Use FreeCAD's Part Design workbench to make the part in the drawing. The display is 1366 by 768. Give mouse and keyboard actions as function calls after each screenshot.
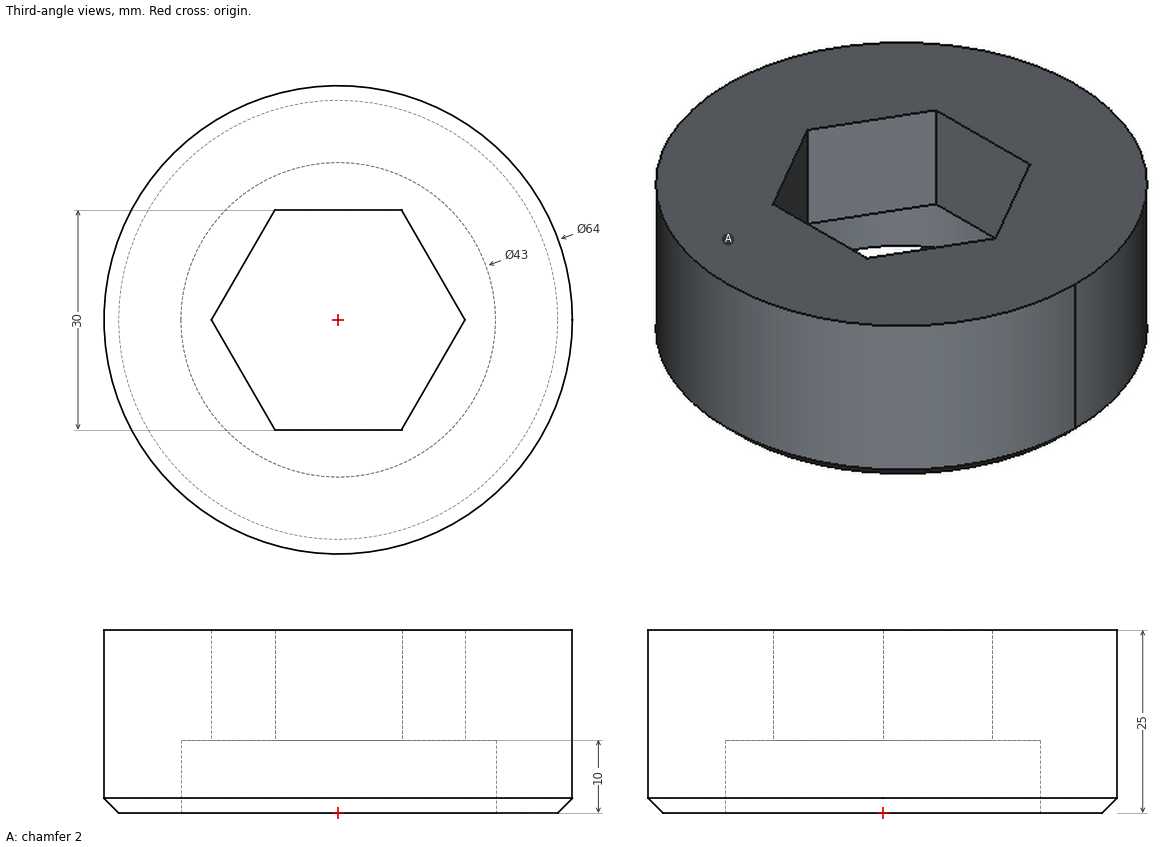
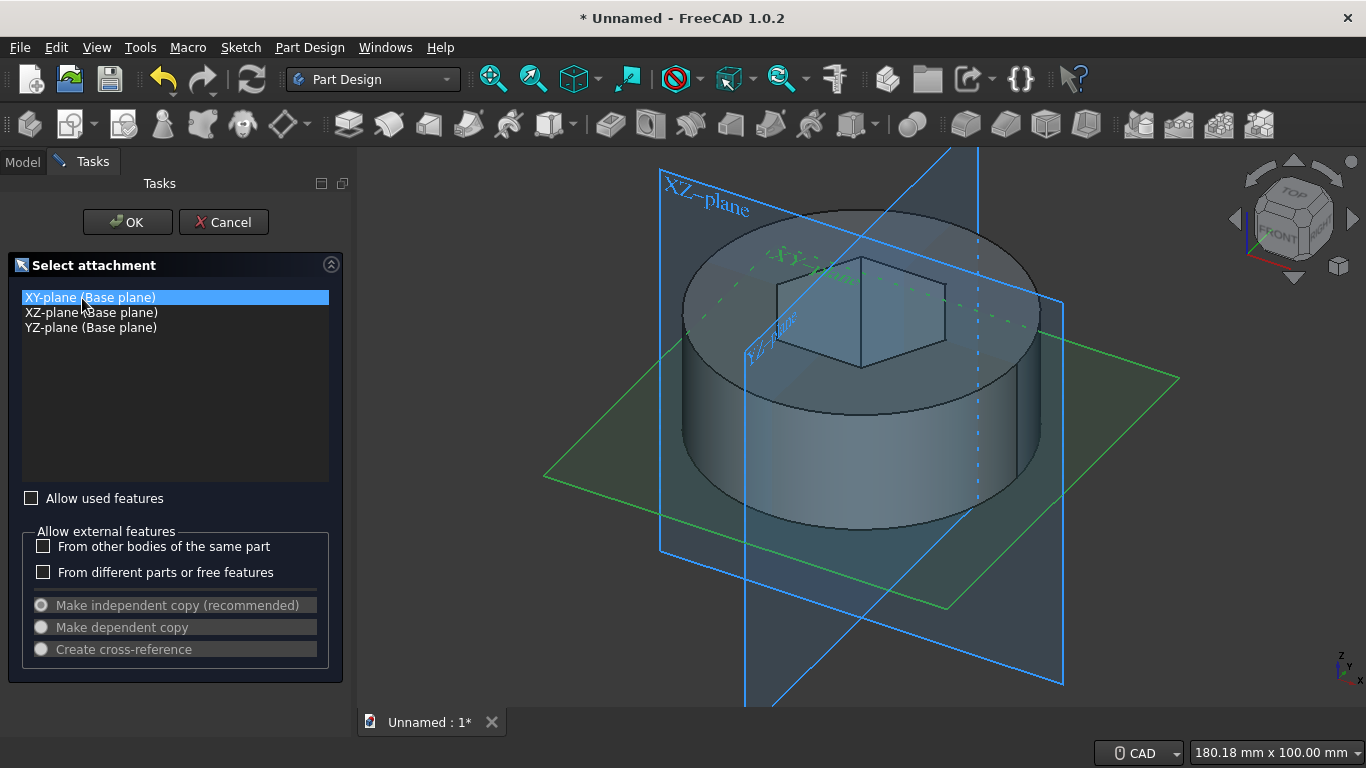
click(128, 222)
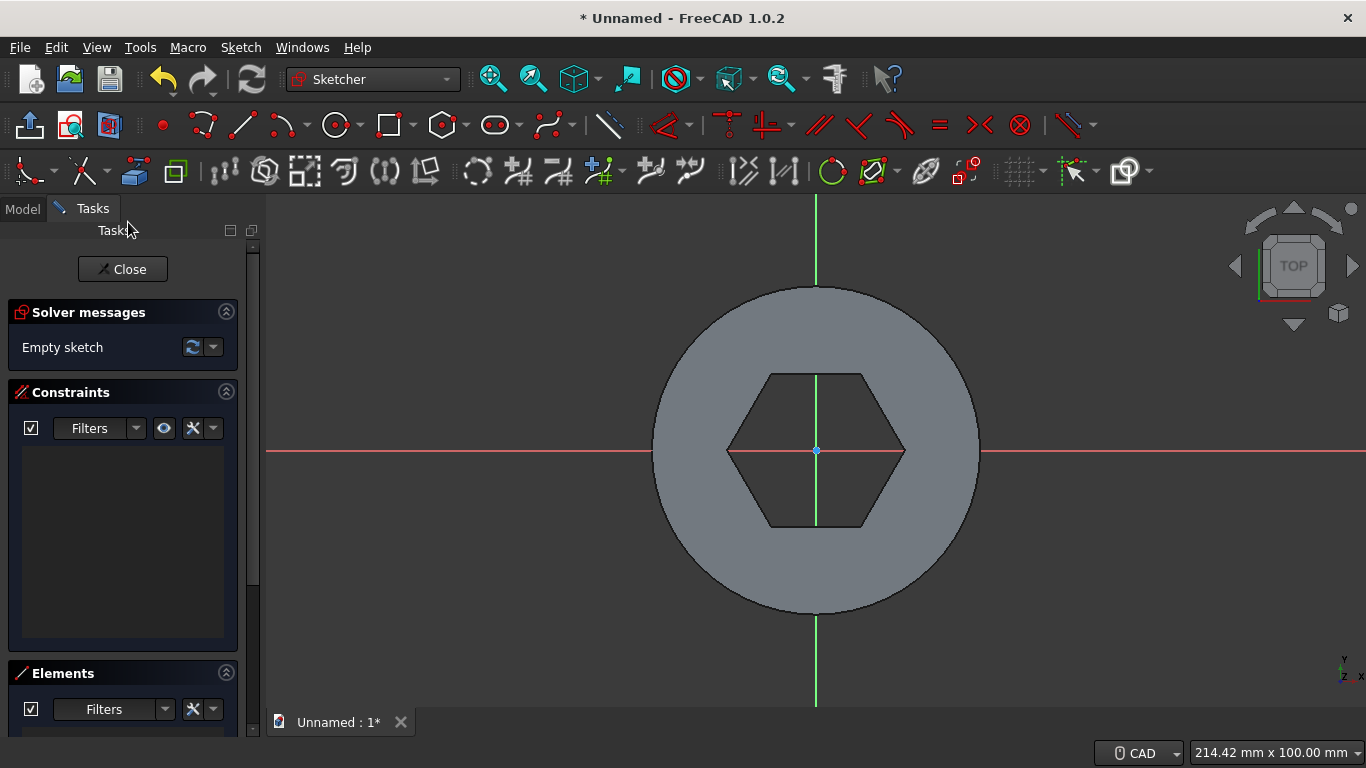
key(q)
key(s)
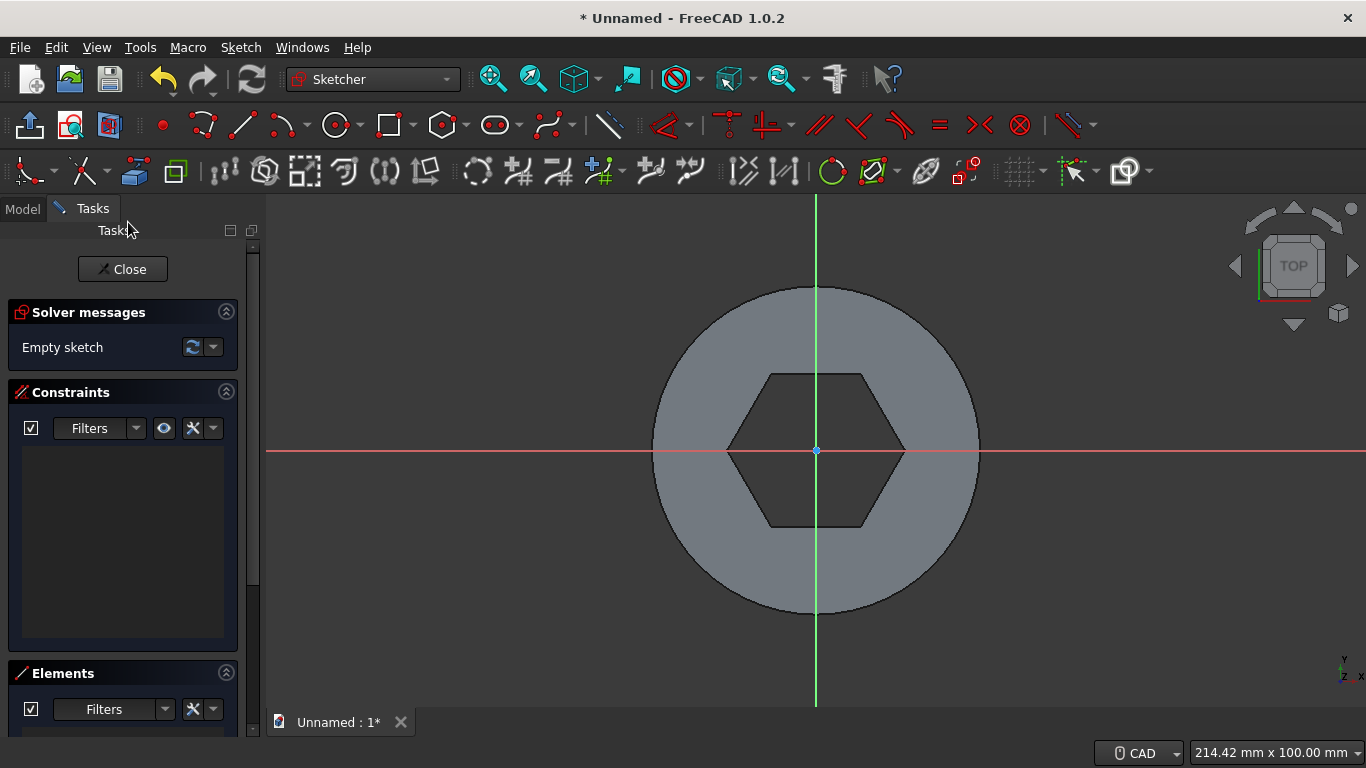
scroll(955, 451, up, 2)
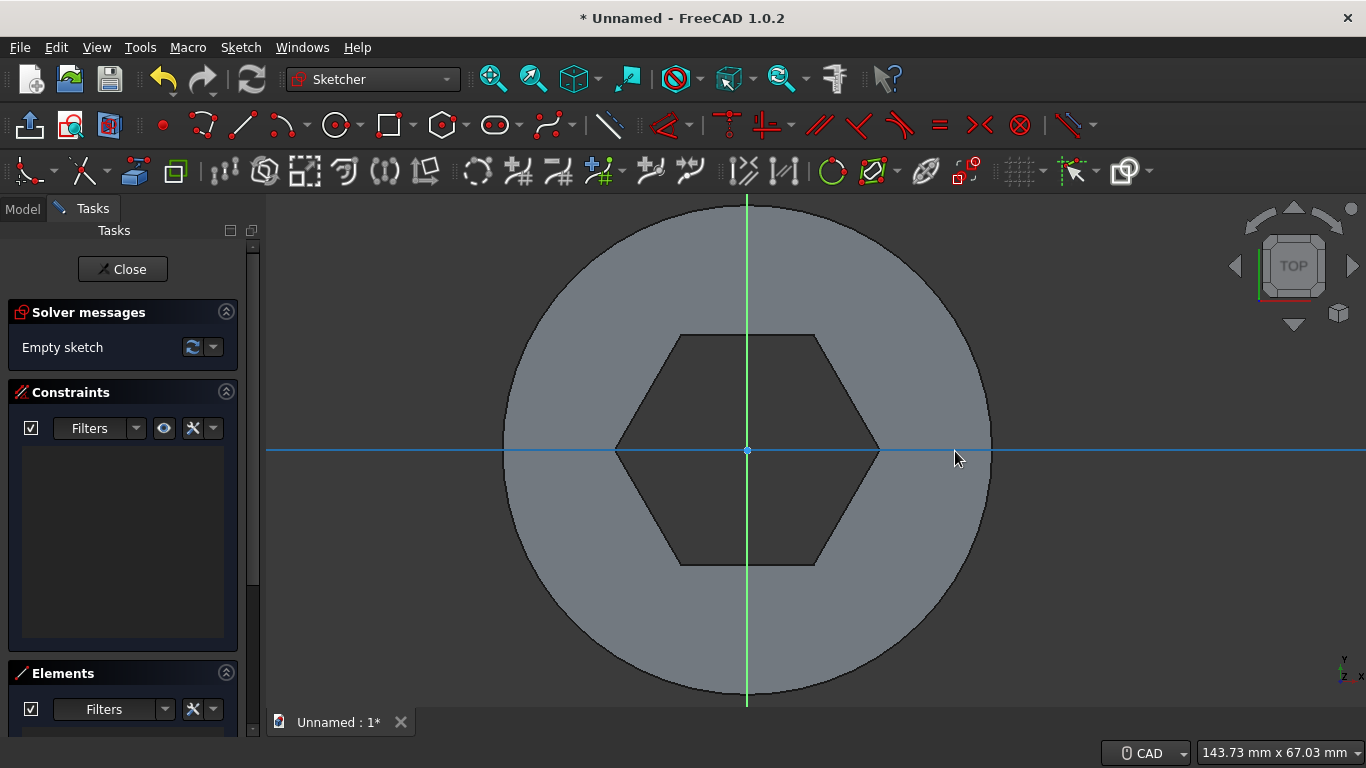
key(g)
key(c)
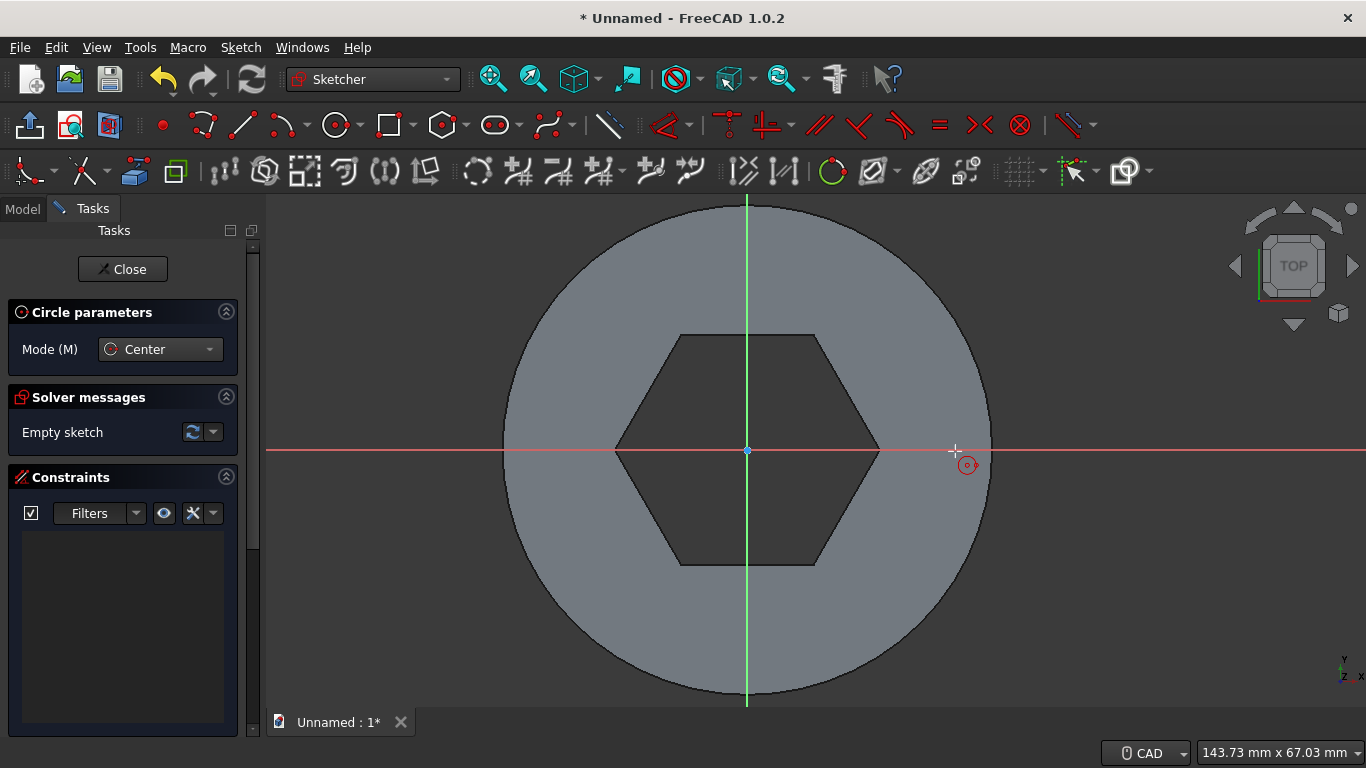
click(747, 450)
click(864, 334)
key(Escape)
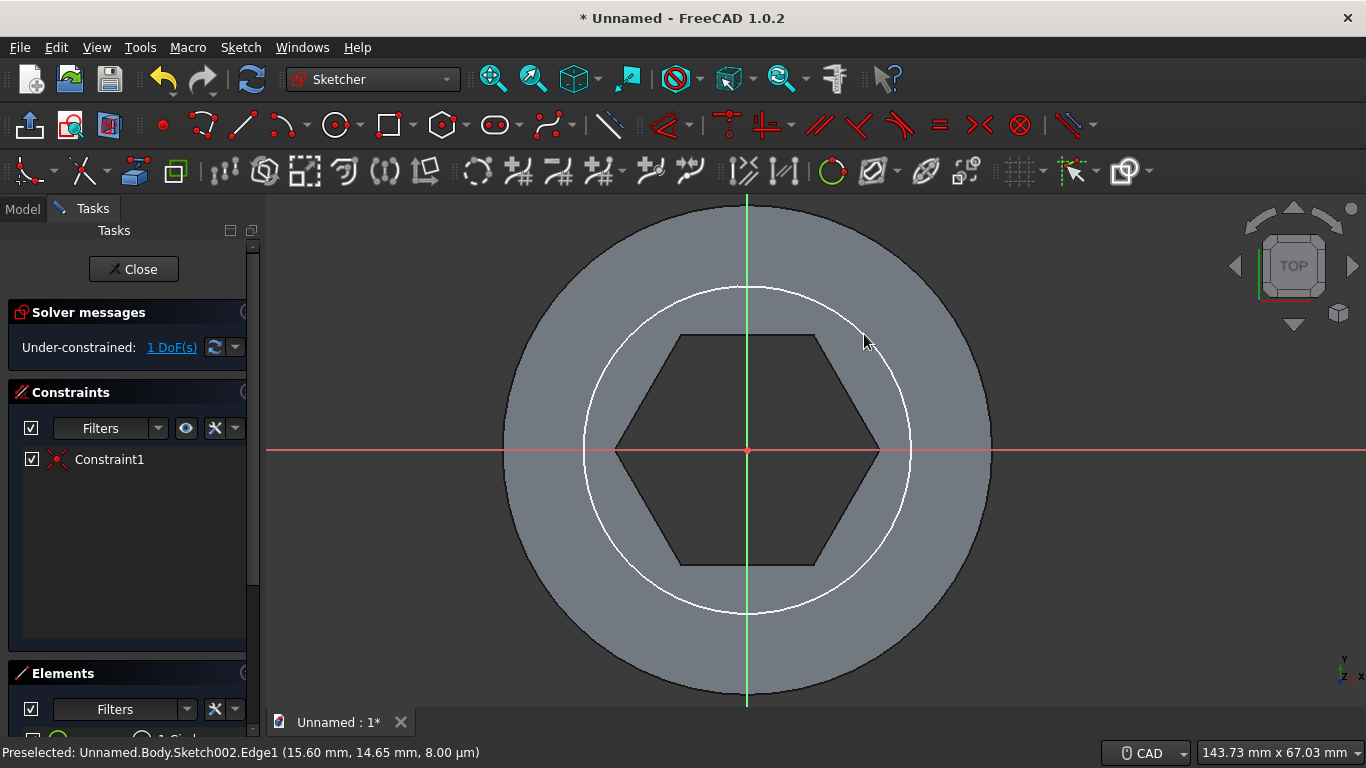
click(664, 126)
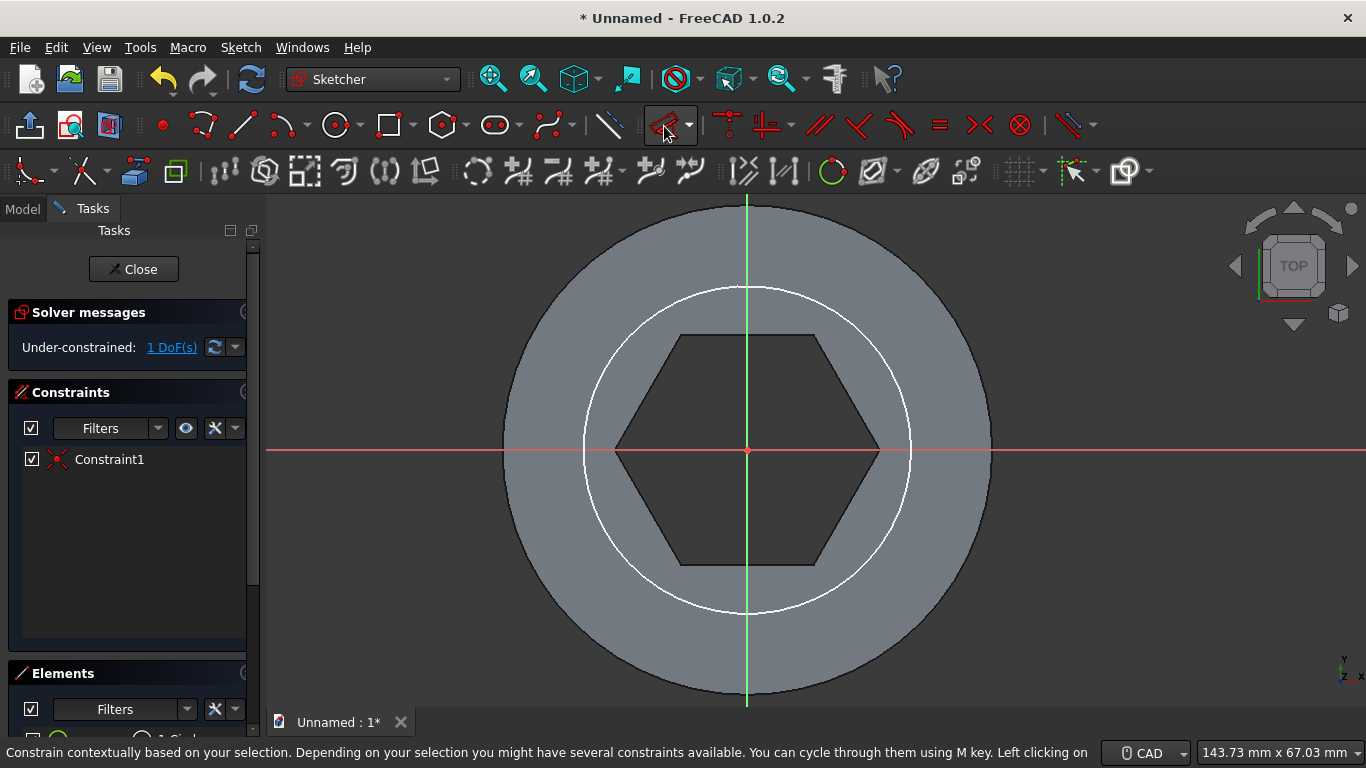
click(863, 334)
click(886, 311)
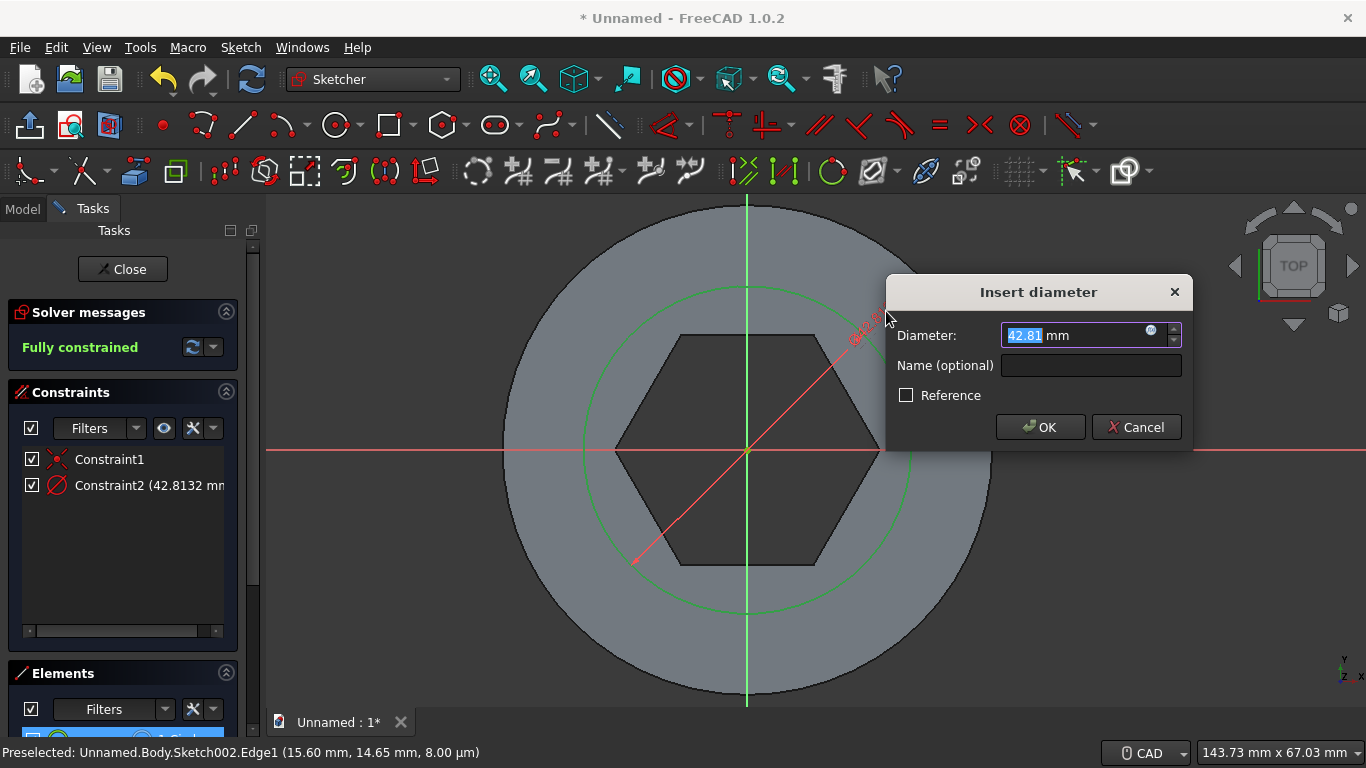
text(43)
key(Return)
key(Escape)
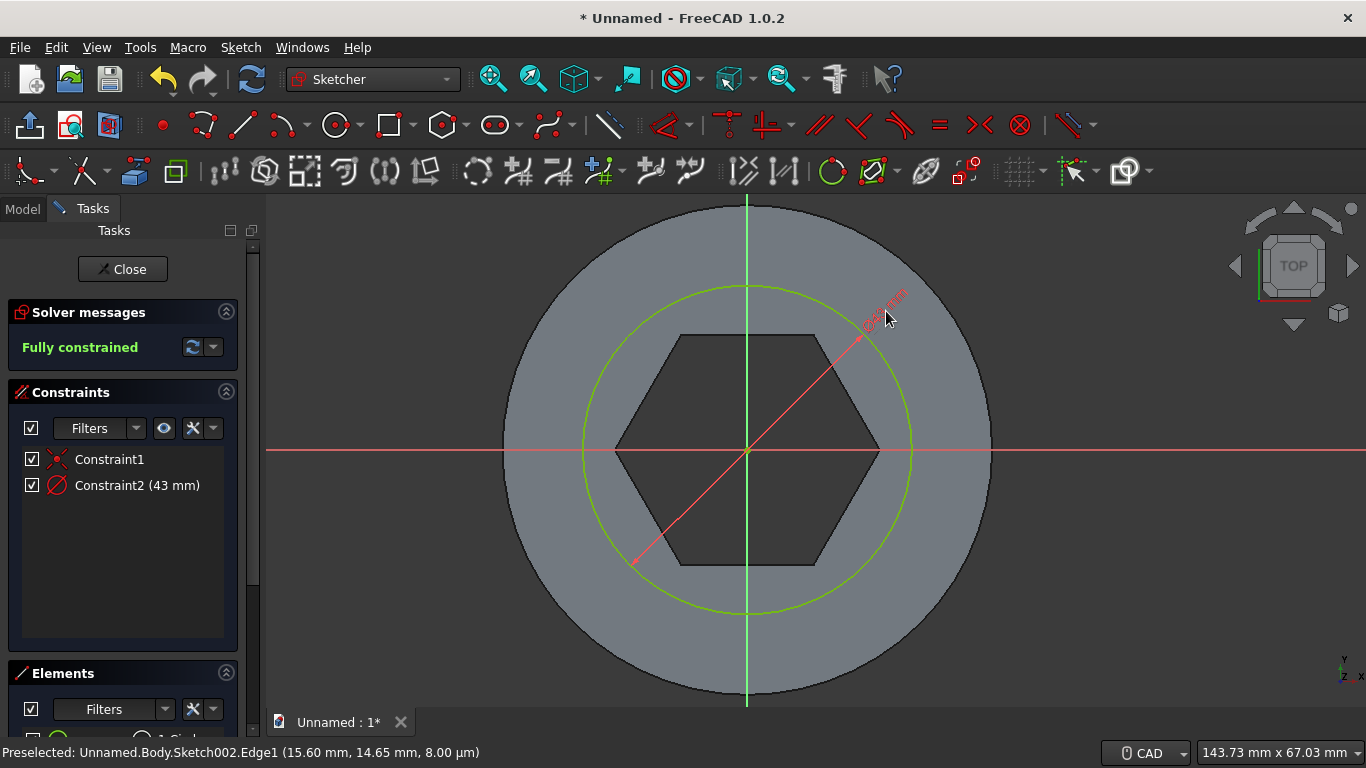
click(123, 269)